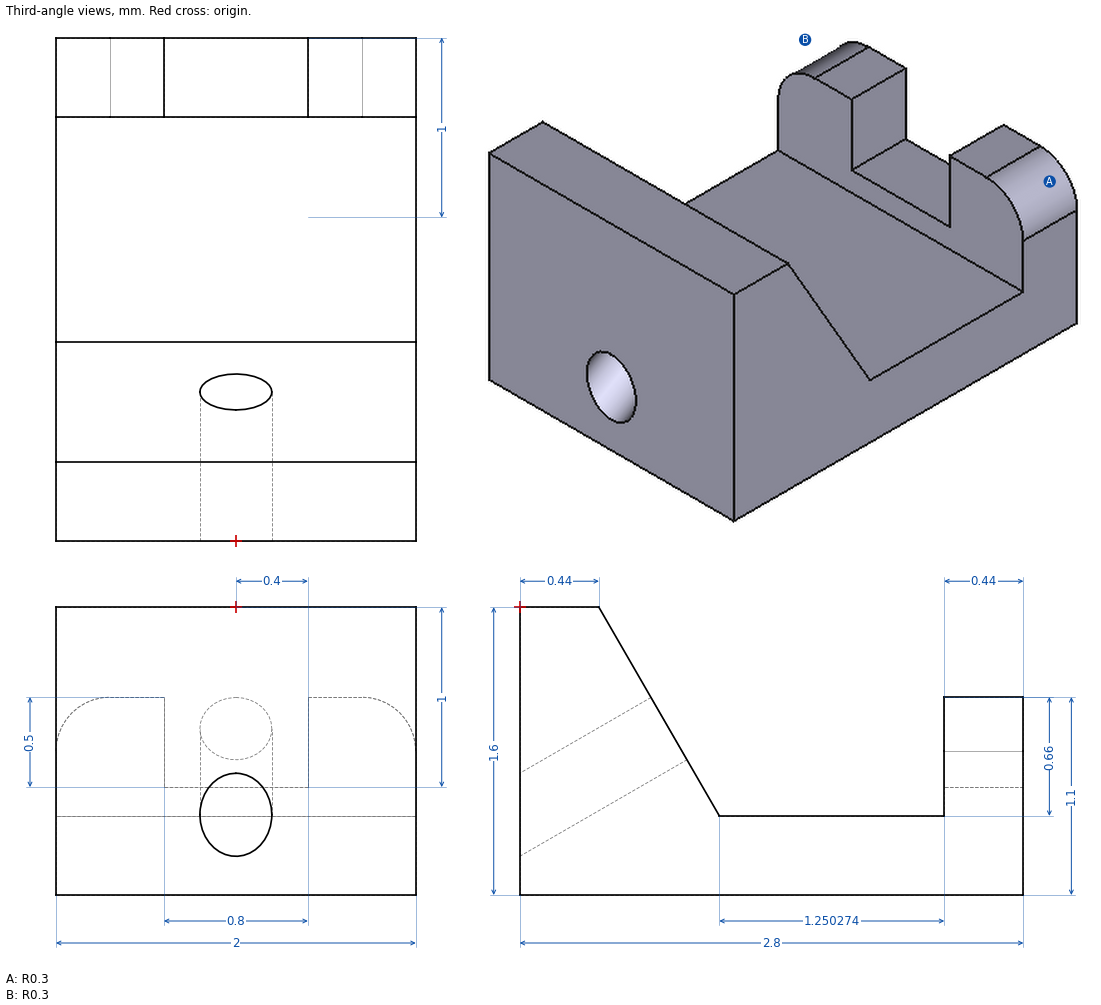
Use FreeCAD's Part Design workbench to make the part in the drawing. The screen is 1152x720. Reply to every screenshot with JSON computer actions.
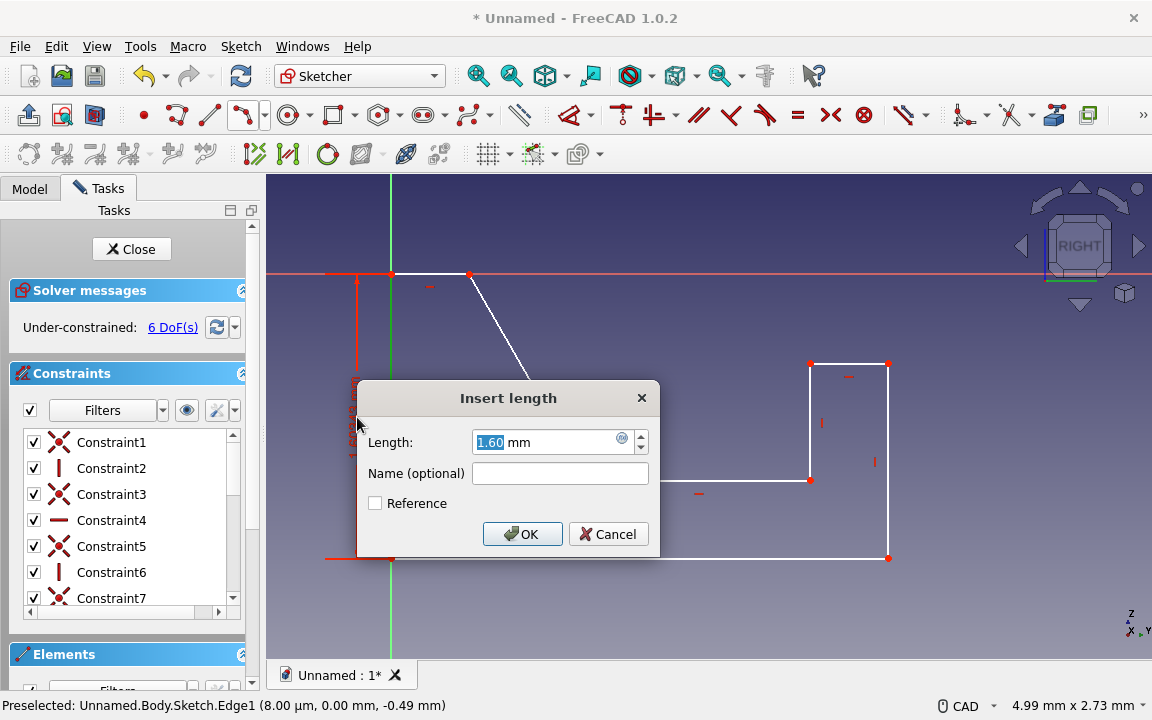
{"action": "type", "text": "1.6"}
{"action": "key", "text": "Return"}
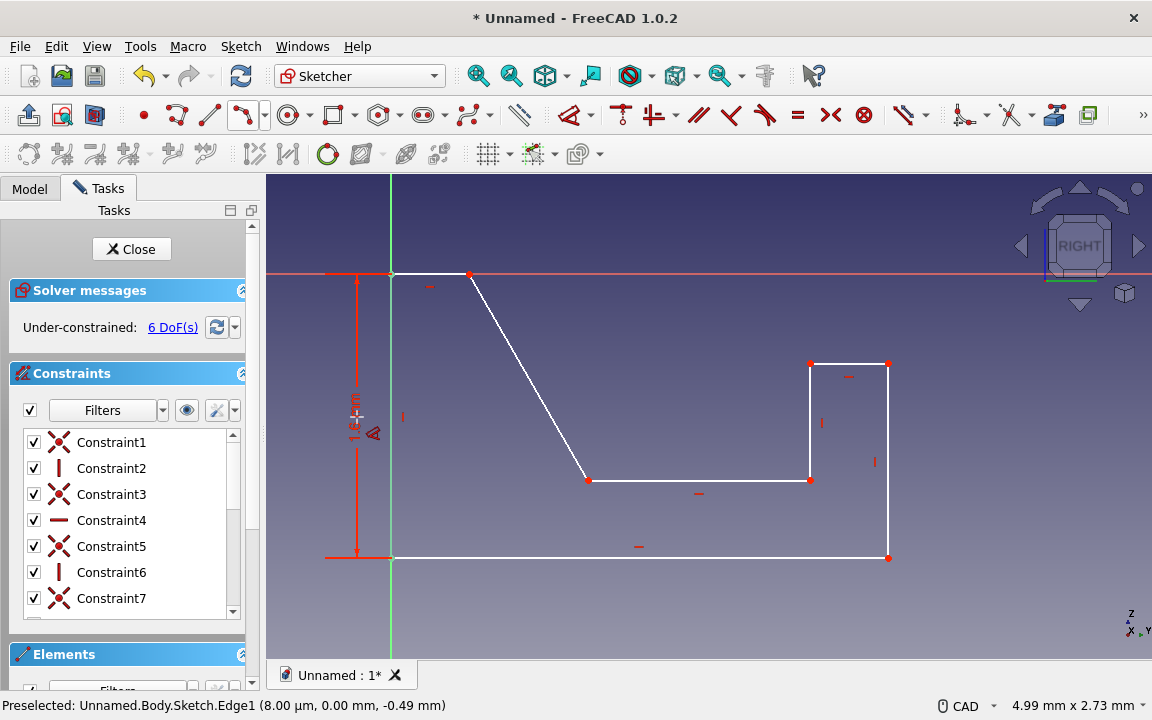
{"action": "left_click", "coordinate": [540, 558]}
{"action": "left_click", "coordinate": [640, 592]}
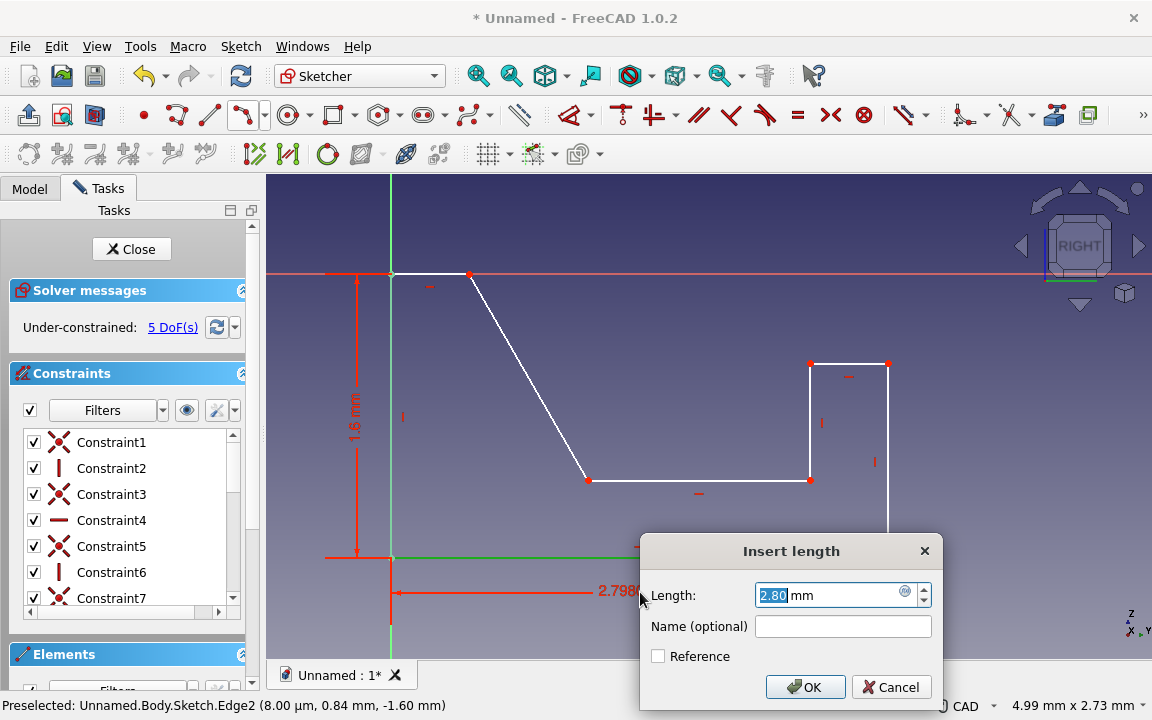
{"action": "type", "text": "2.8"}
{"action": "key", "text": "Return"}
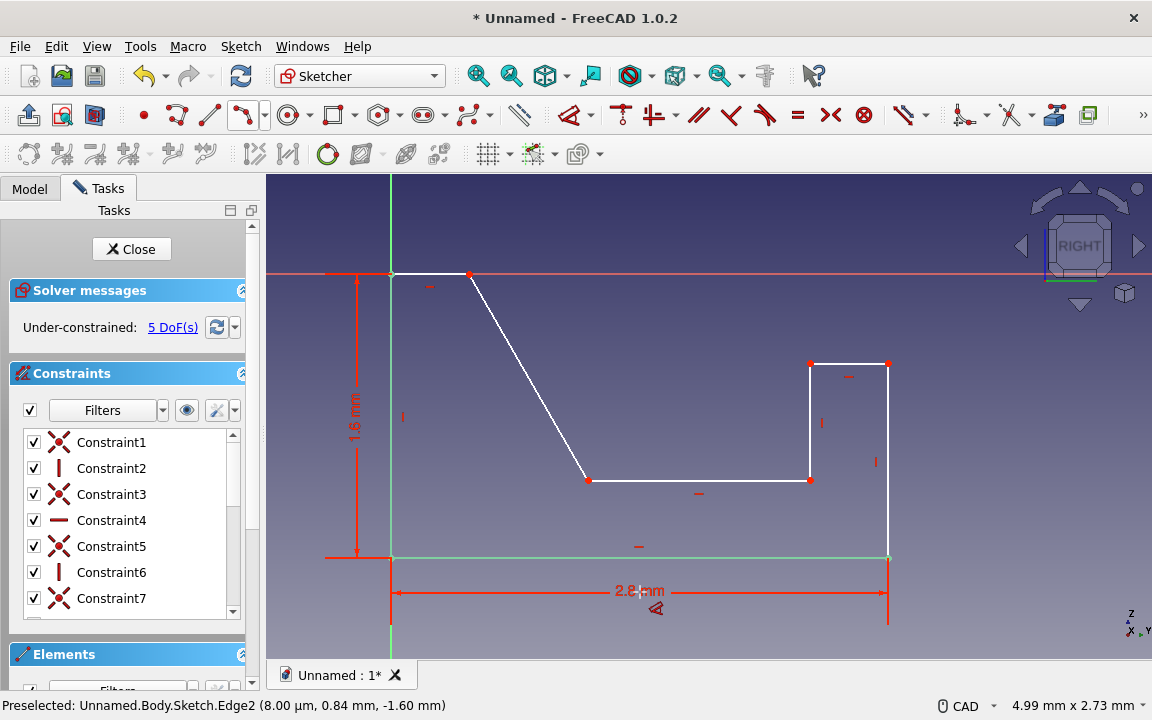
{"action": "left_click", "coordinate": [888, 500]}
{"action": "left_click", "coordinate": [922, 461]}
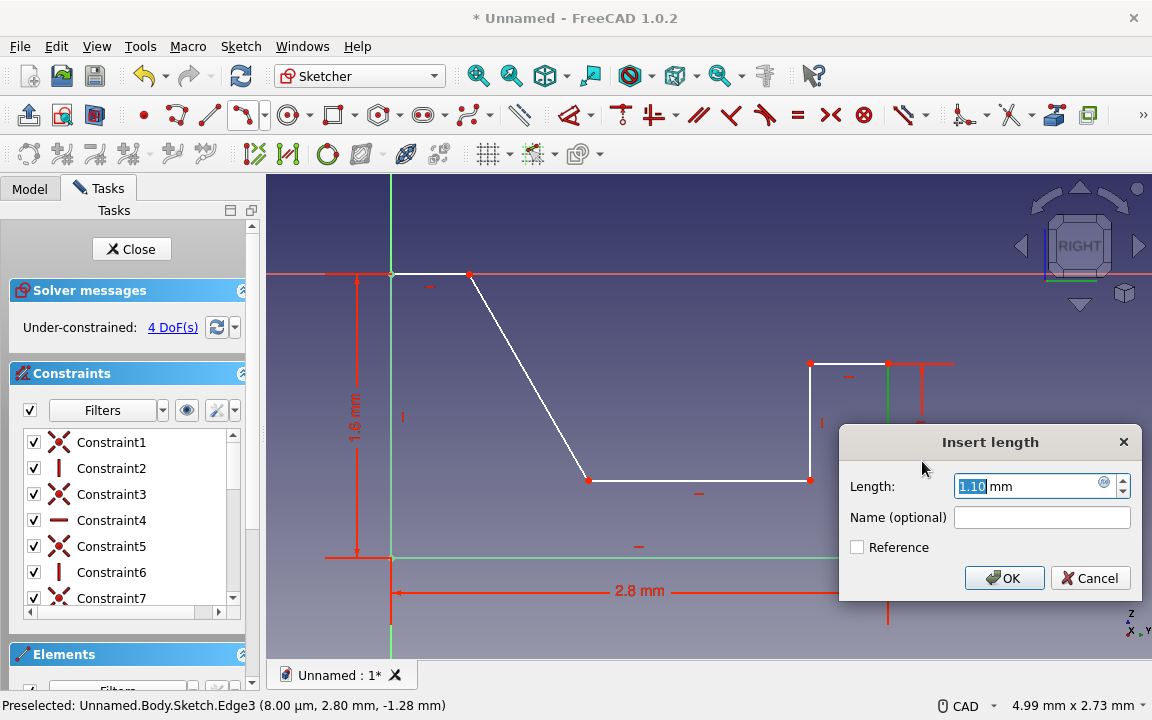
{"action": "type", "text": "1.1"}
{"action": "key", "text": "Return"}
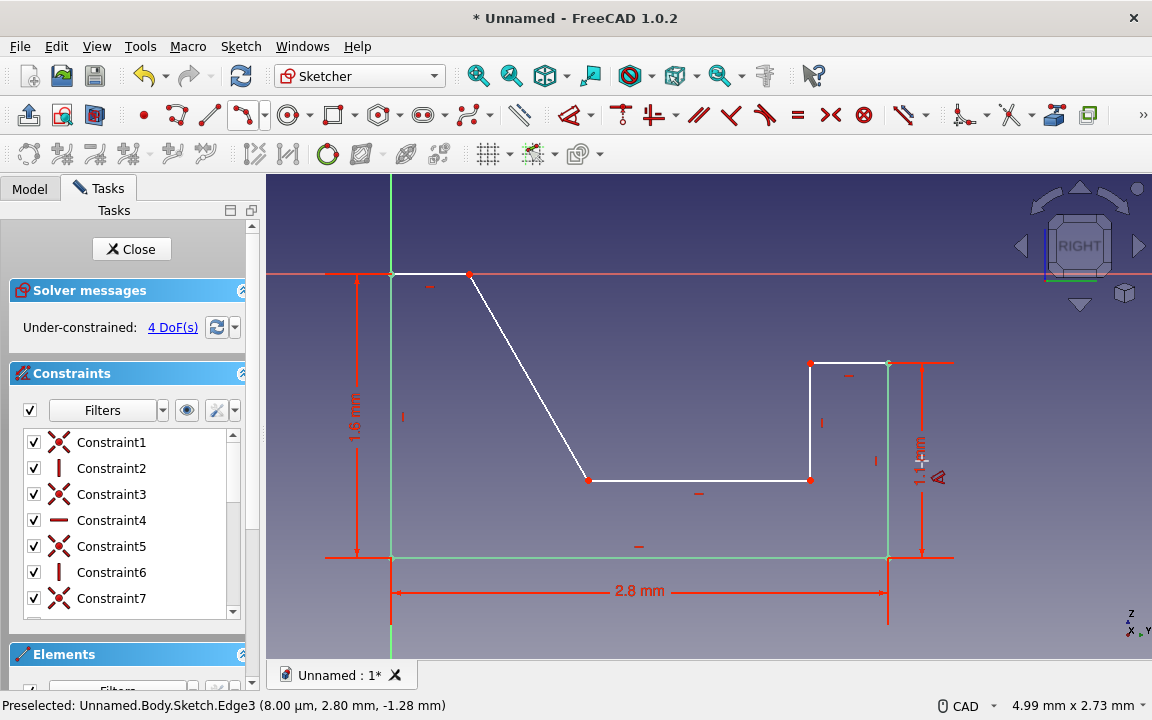
{"action": "left_click", "coordinate": [865, 363]}
{"action": "left_click", "coordinate": [849, 329]}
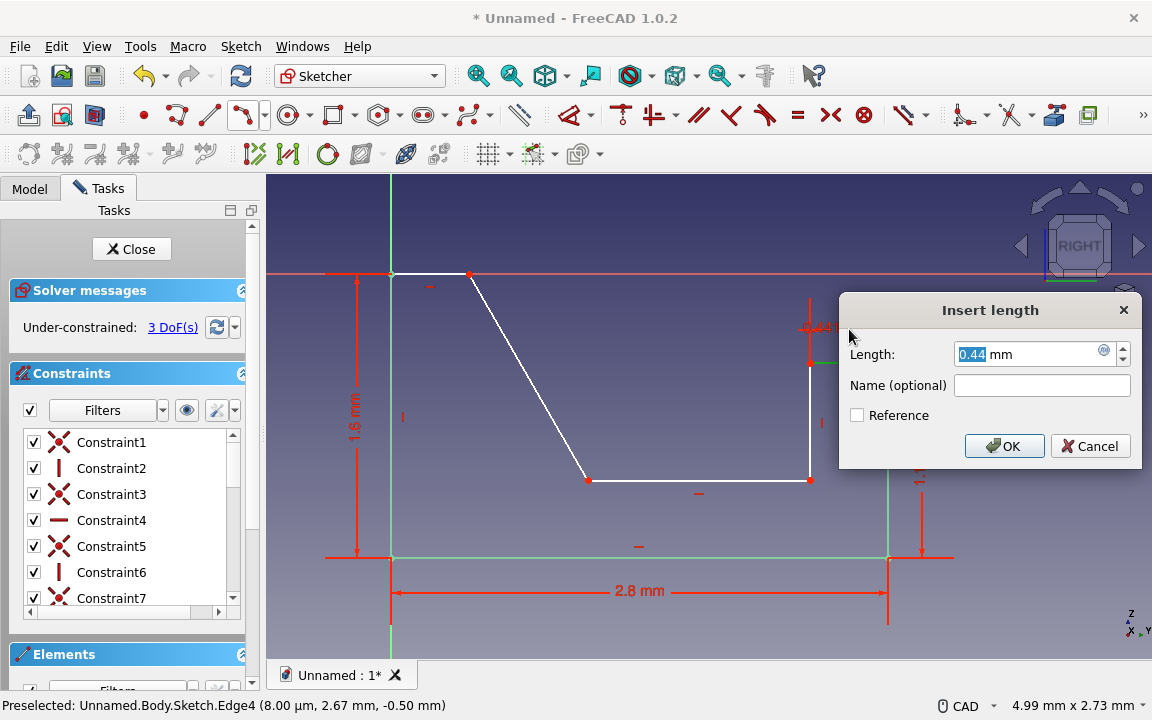
{"action": "type", "text": "0.44"}
{"action": "key", "text": "Return"}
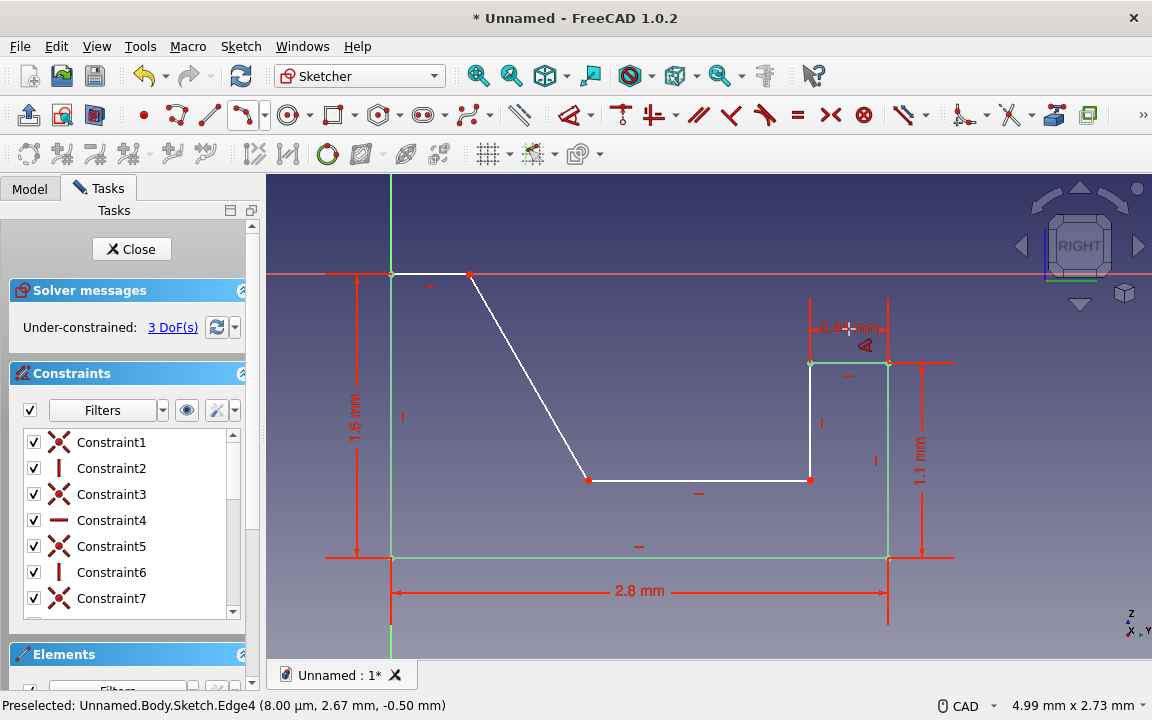
{"action": "left_click", "coordinate": [810, 398]}
{"action": "left_click", "coordinate": [844, 422]}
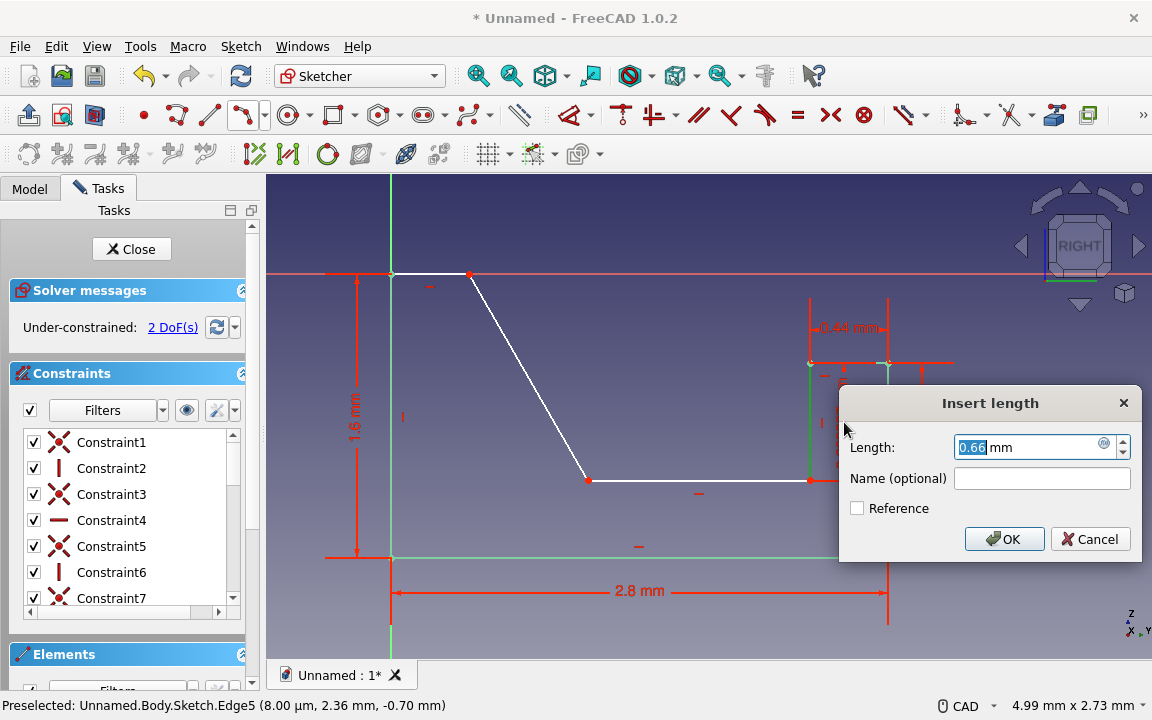
{"action": "type", "text": "0.66"}
{"action": "key", "text": "Return"}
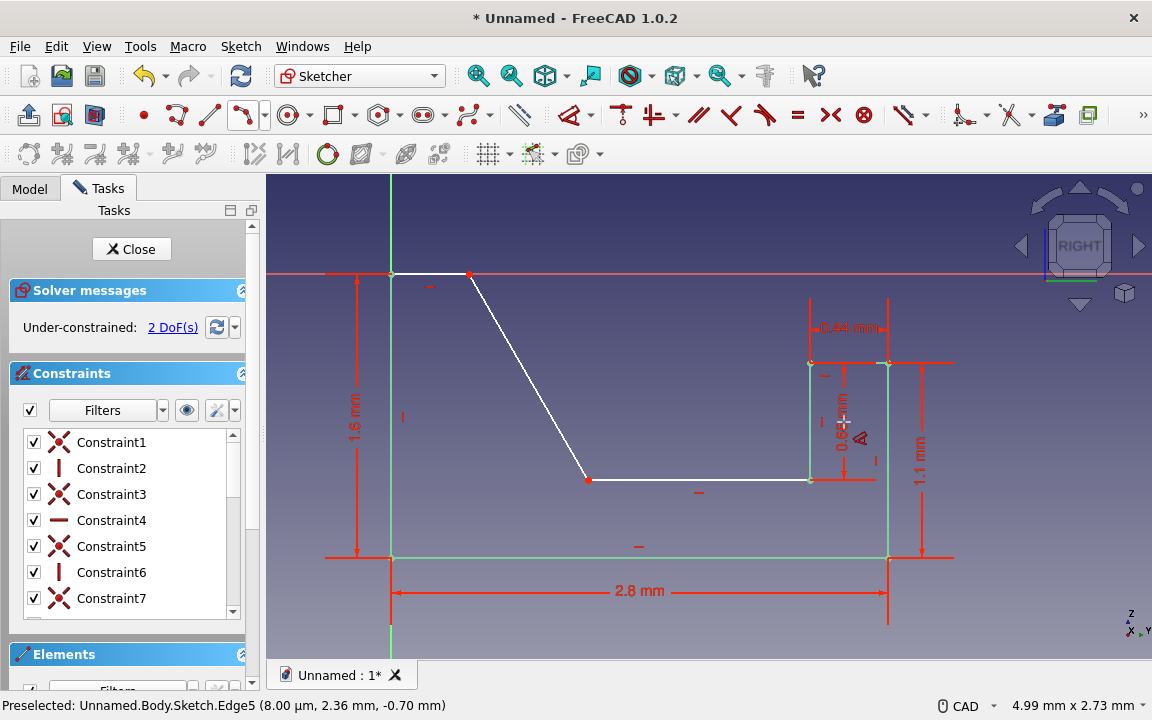
{"action": "left_click", "coordinate": [446, 274]}
{"action": "left_click", "coordinate": [430, 240]}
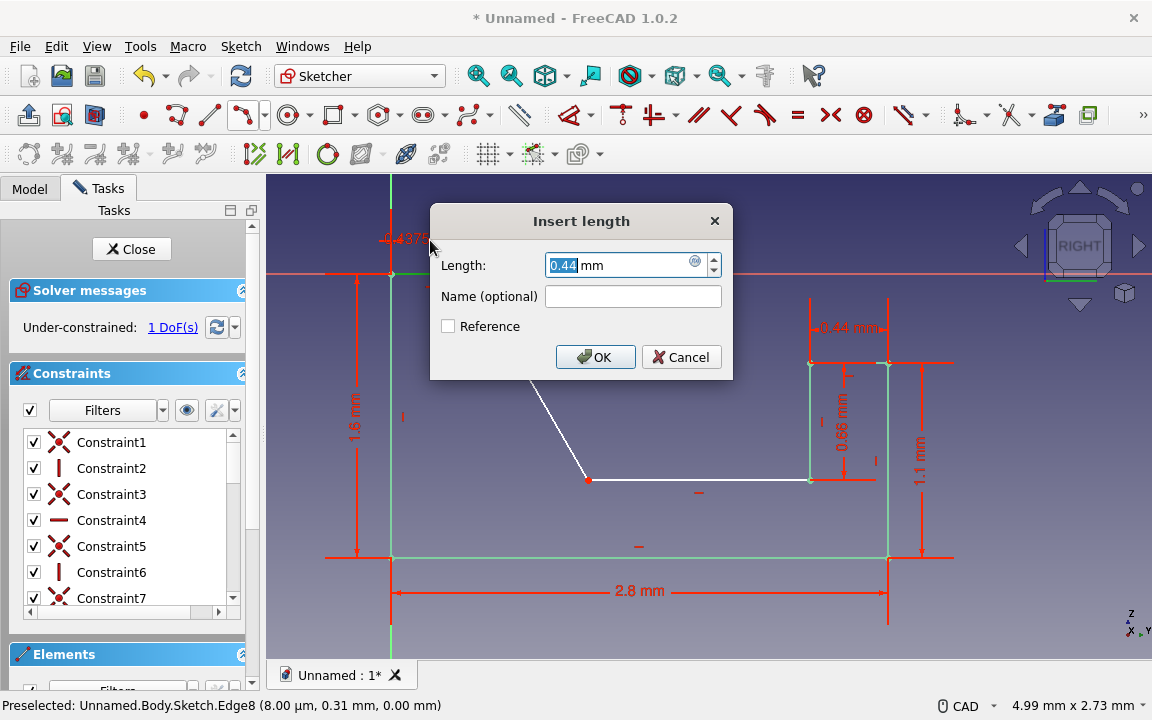
{"action": "type", "text": "0.44"}
{"action": "key", "text": "Return"}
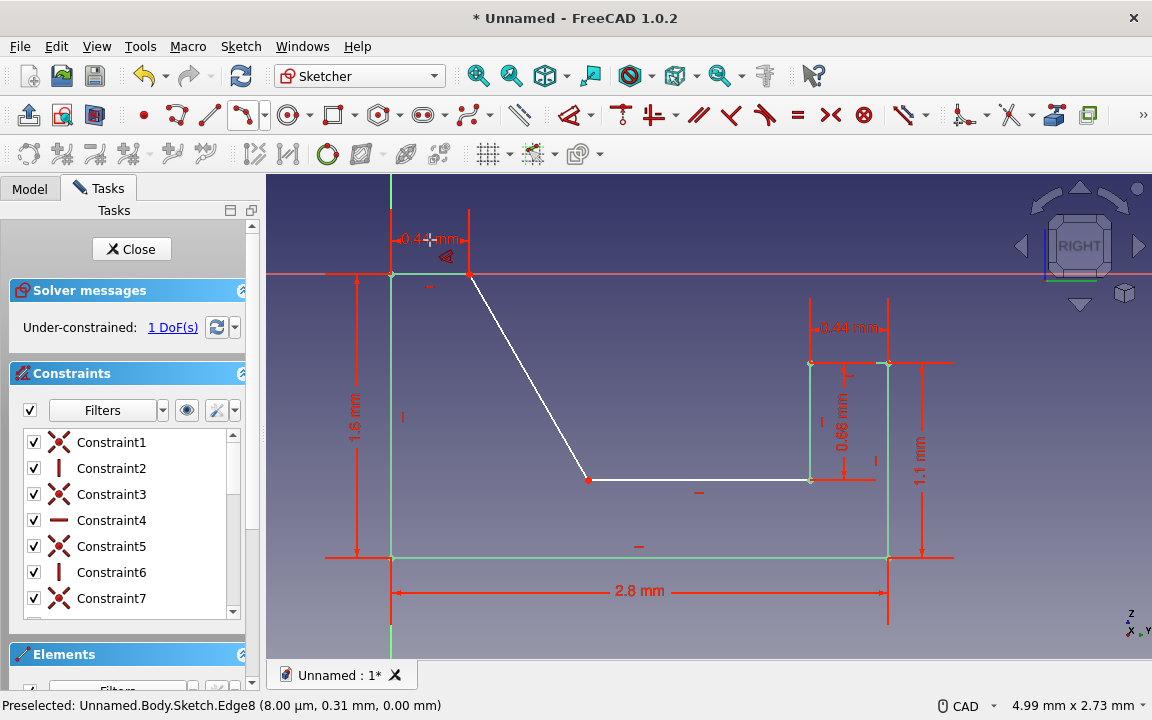
{"action": "left_click", "coordinate": [744, 480]}
{"action": "left_click", "coordinate": [699, 514]}